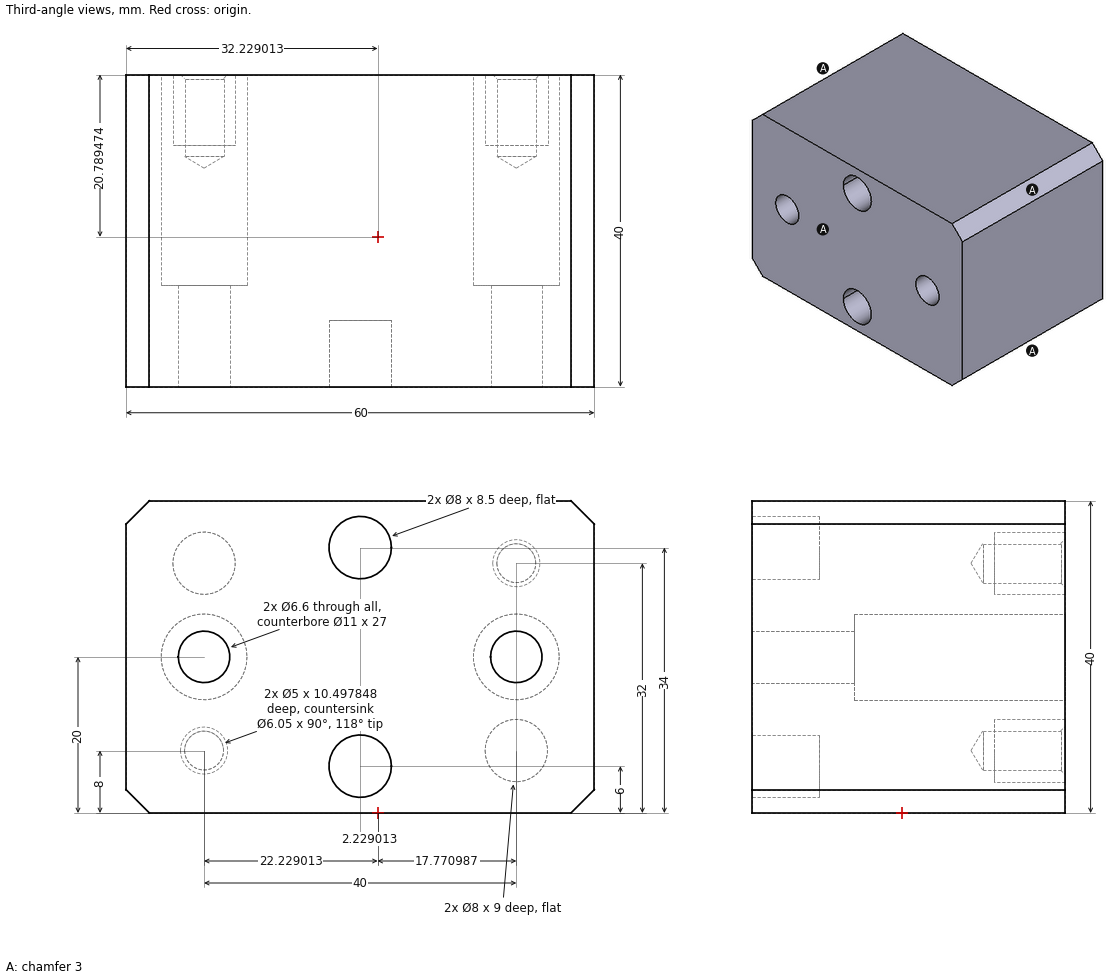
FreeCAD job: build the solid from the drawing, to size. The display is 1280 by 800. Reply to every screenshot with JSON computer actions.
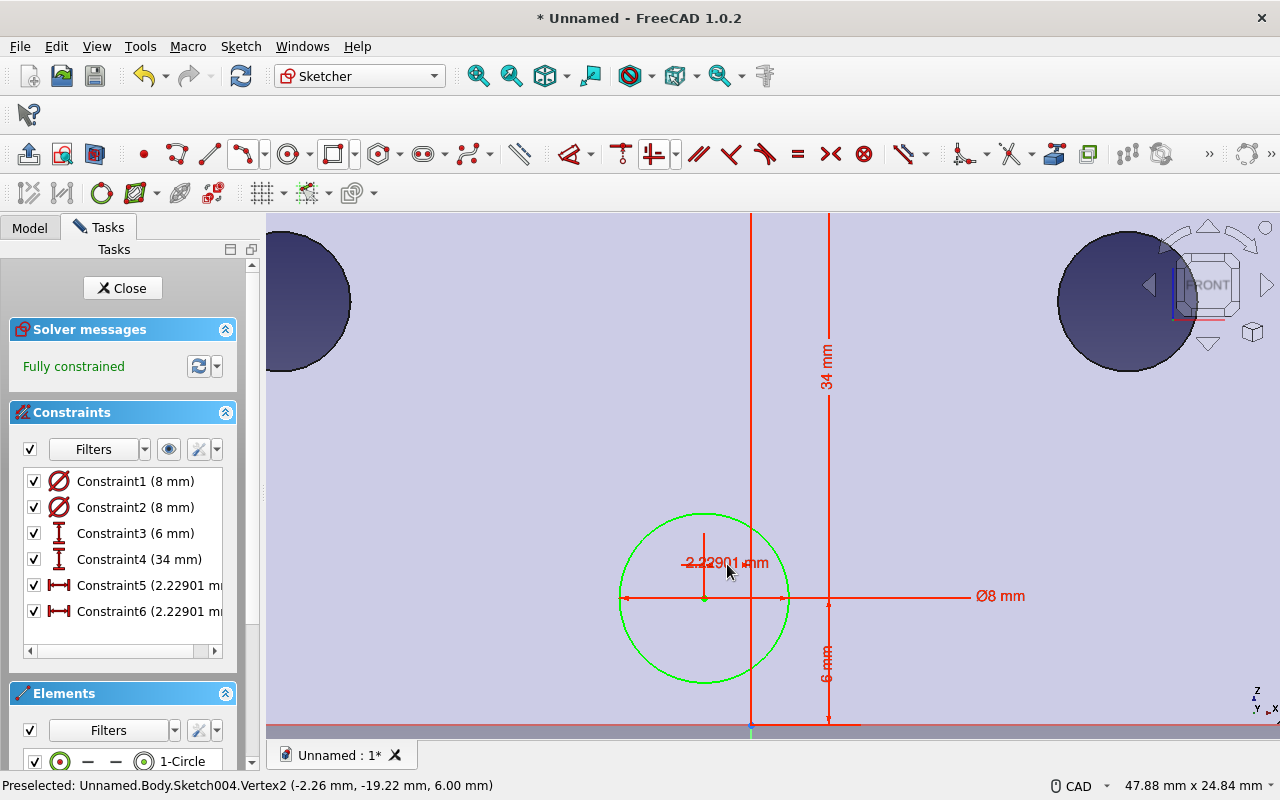
{"action": "left_click", "coordinate": [123, 288]}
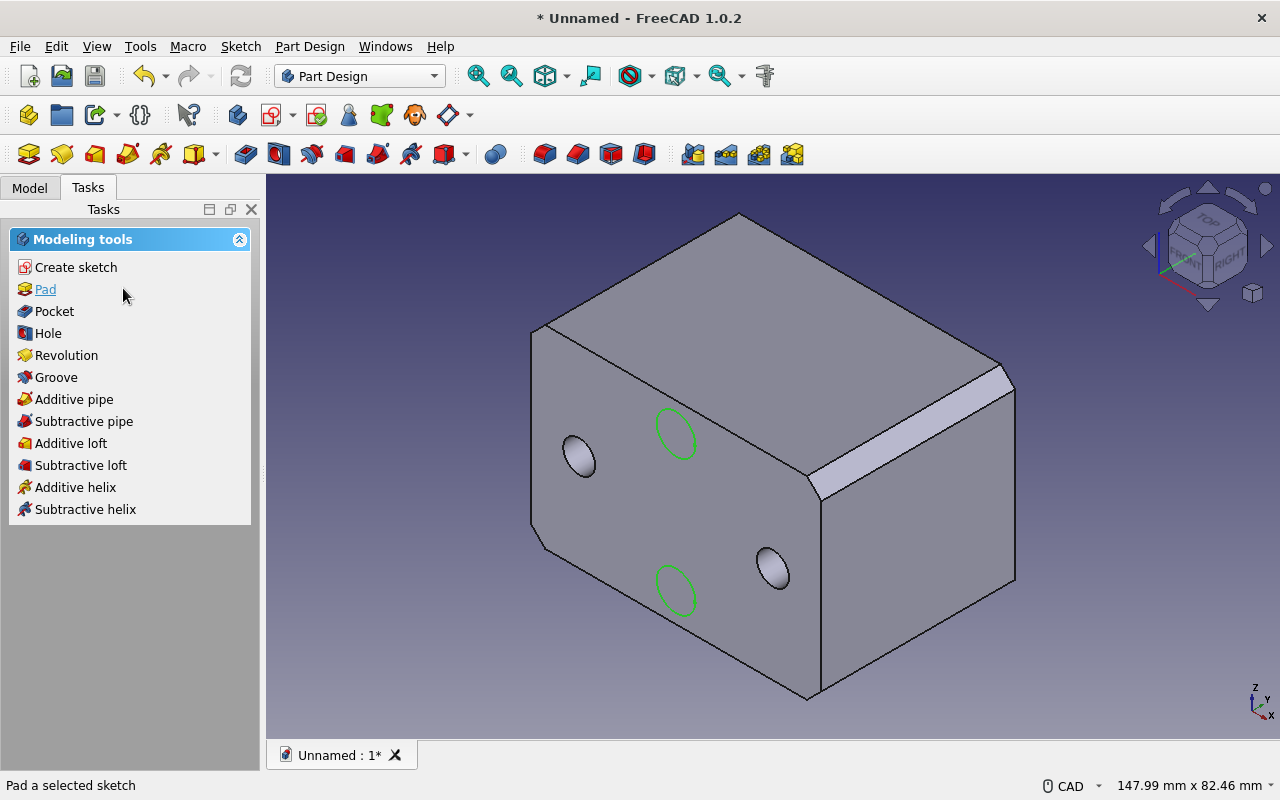
{"action": "left_click", "coordinate": [279, 154]}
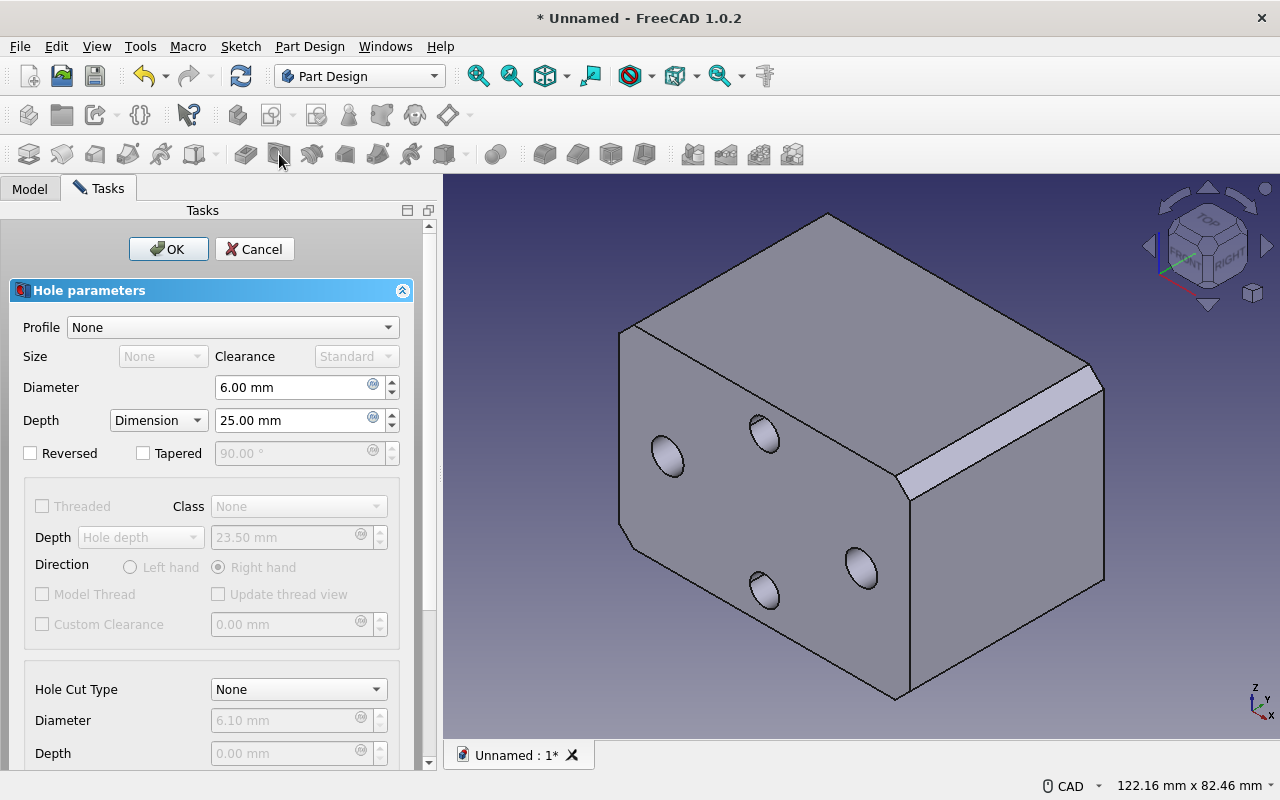
{"action": "triple_click", "coordinate": [300, 388]}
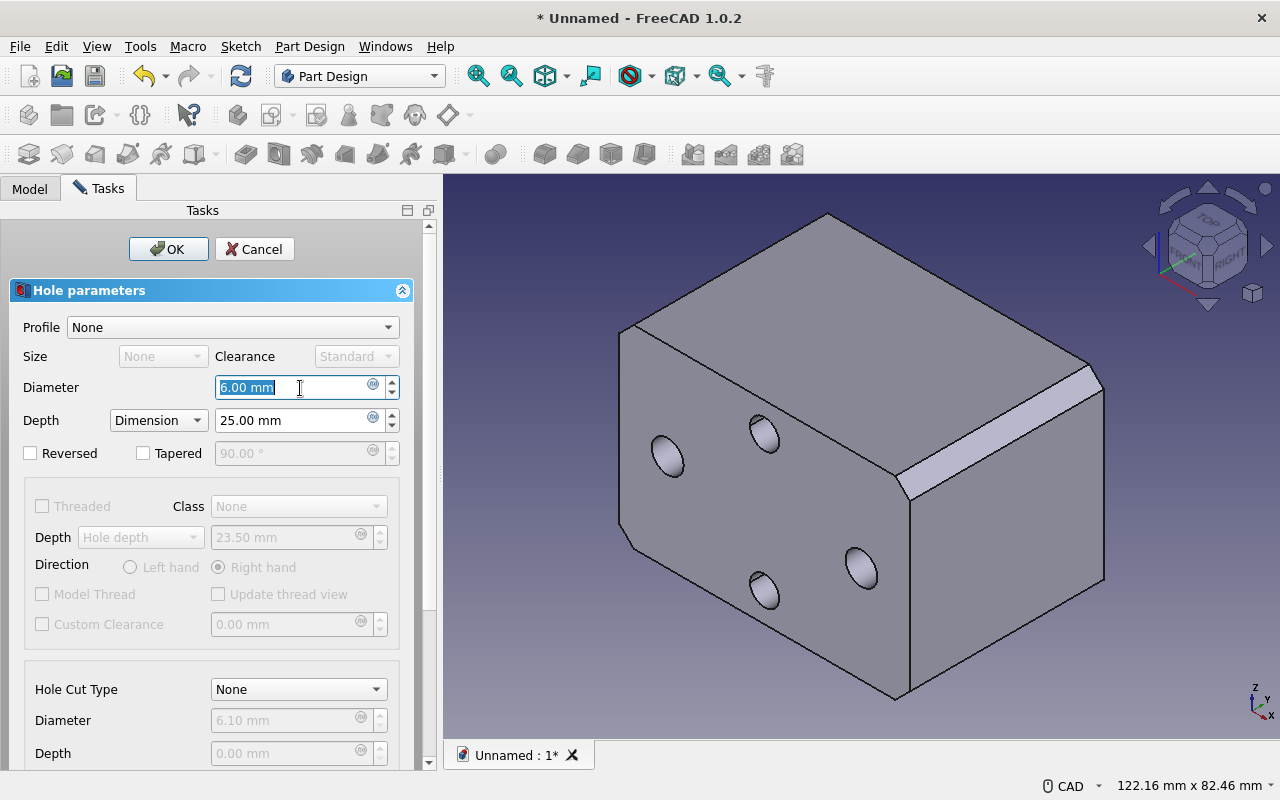
{"action": "type", "text": "8"}
{"action": "key", "text": "Tab"}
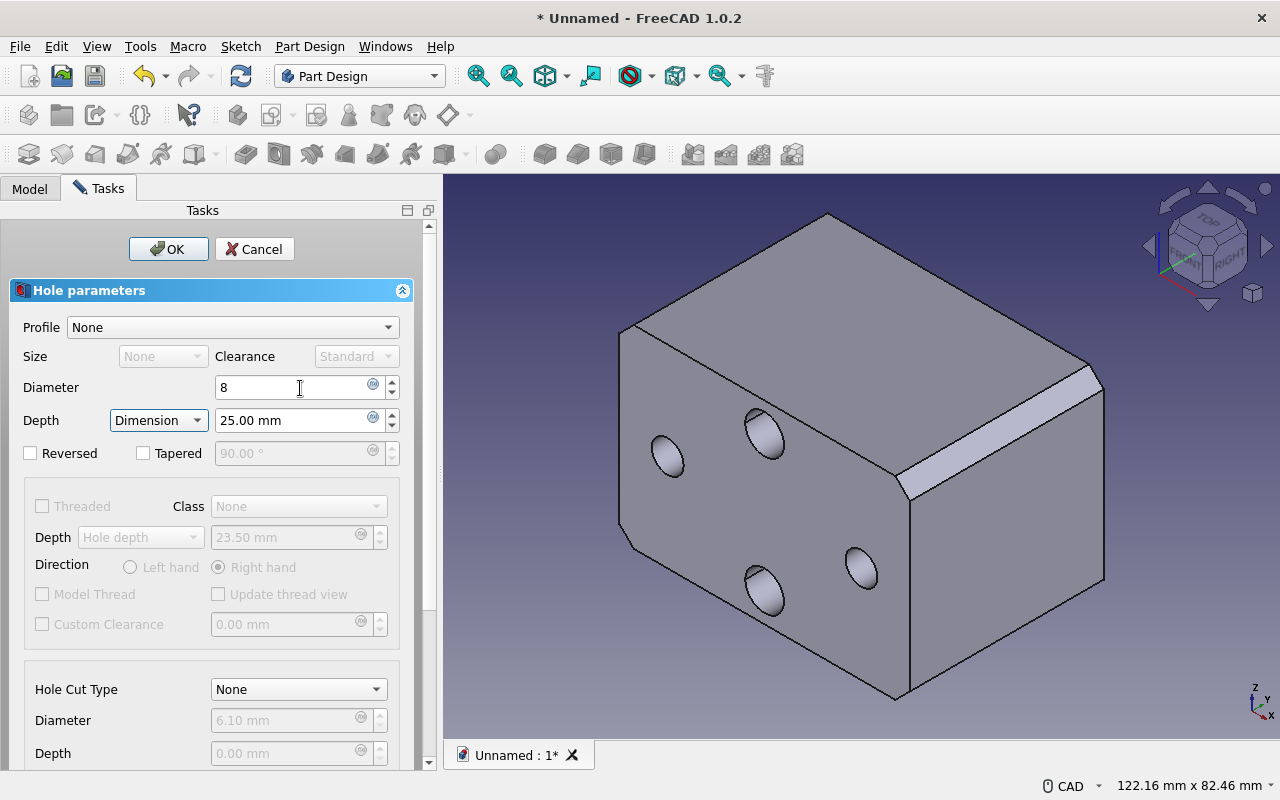
{"action": "triple_click", "coordinate": [300, 420]}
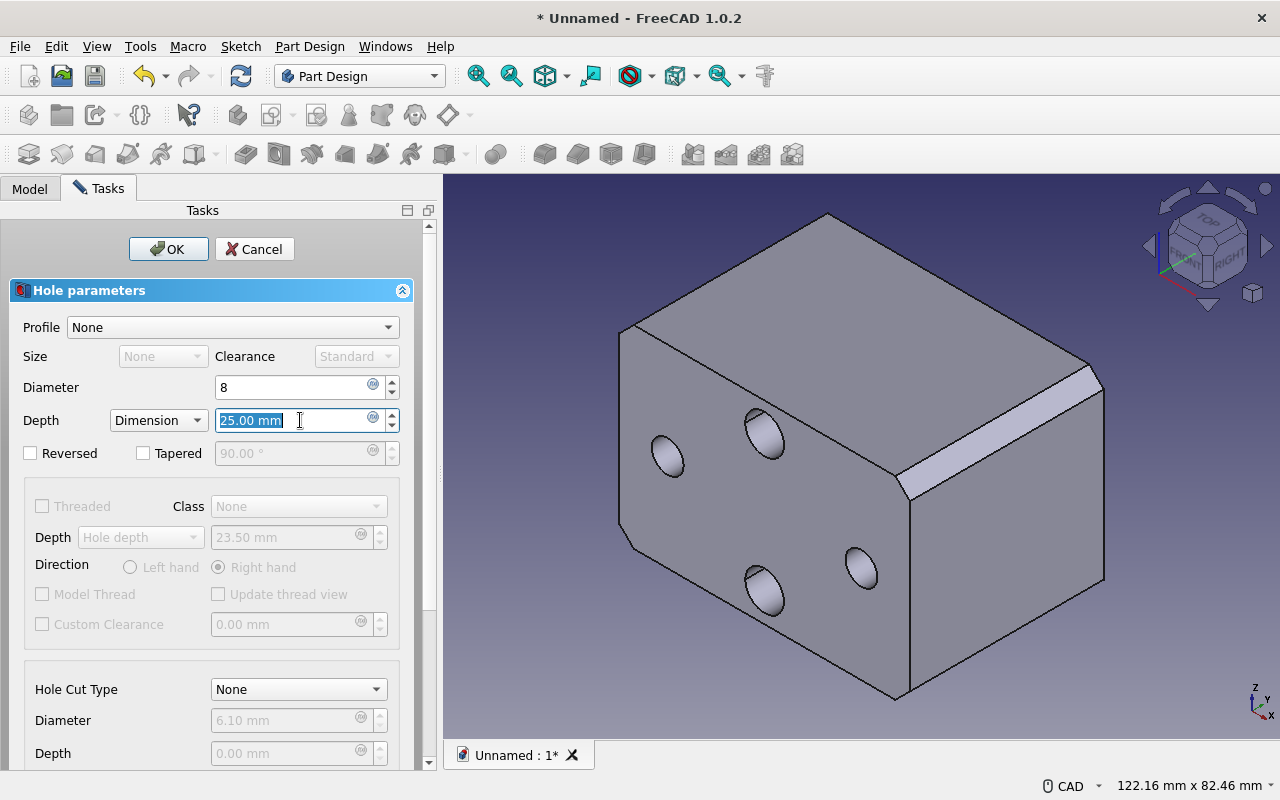
{"action": "type", "text": "8.5"}
{"action": "key", "text": "Tab"}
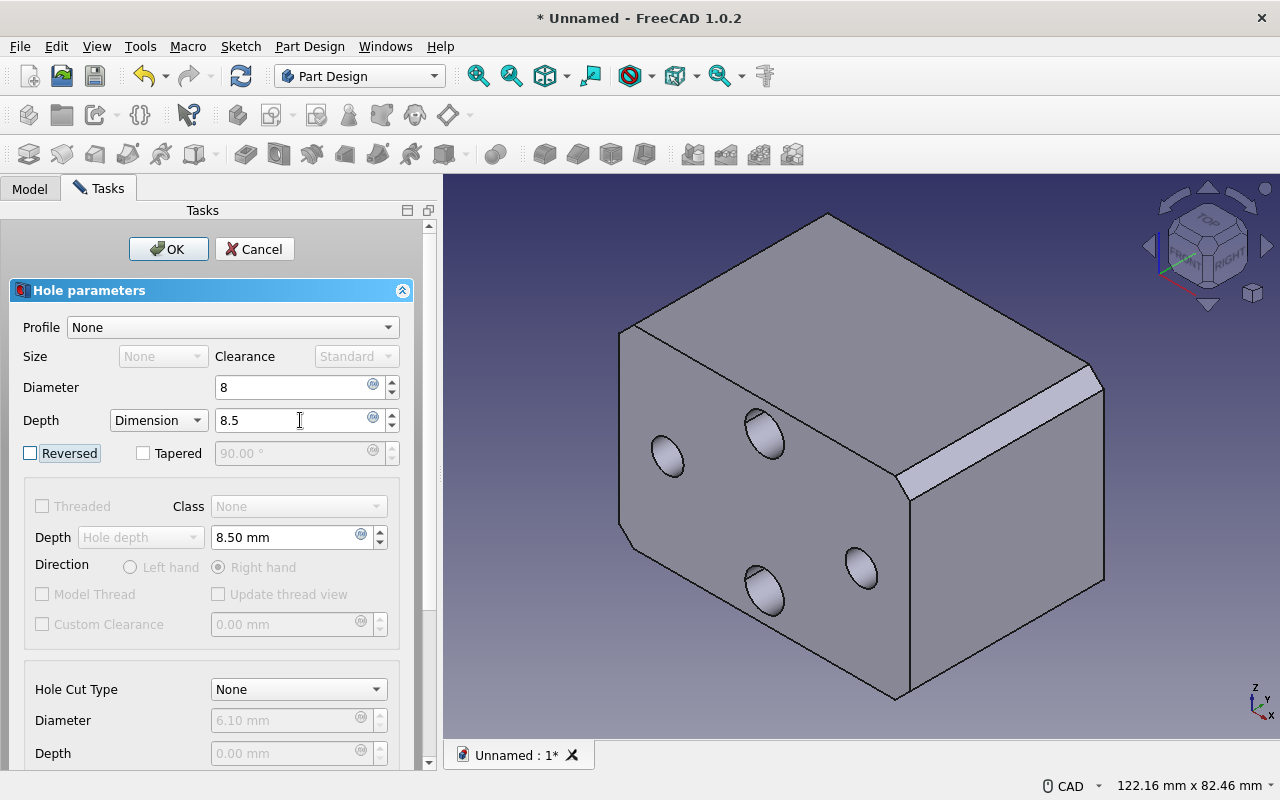
{"action": "scroll", "coordinate": [429, 495], "scroll_direction": "down", "scroll_amount": 3}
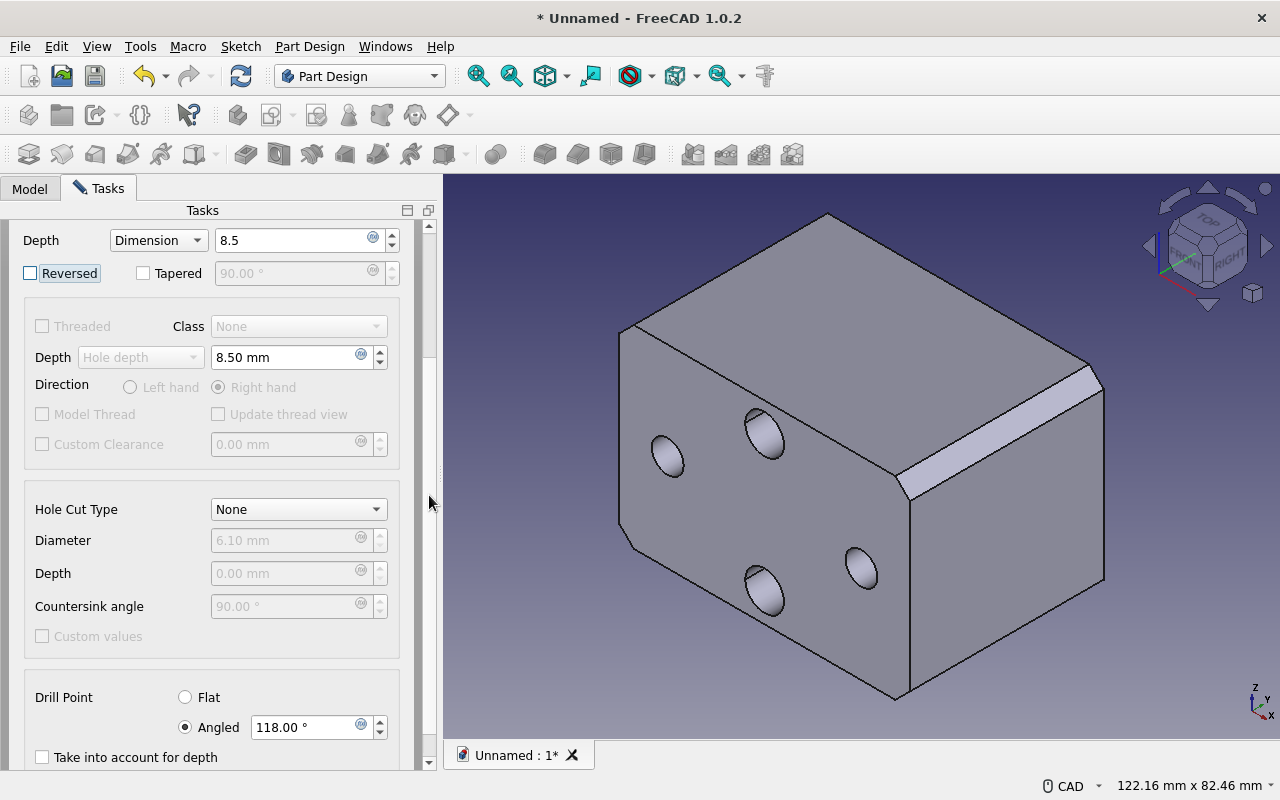
{"action": "left_click", "coordinate": [186, 695]}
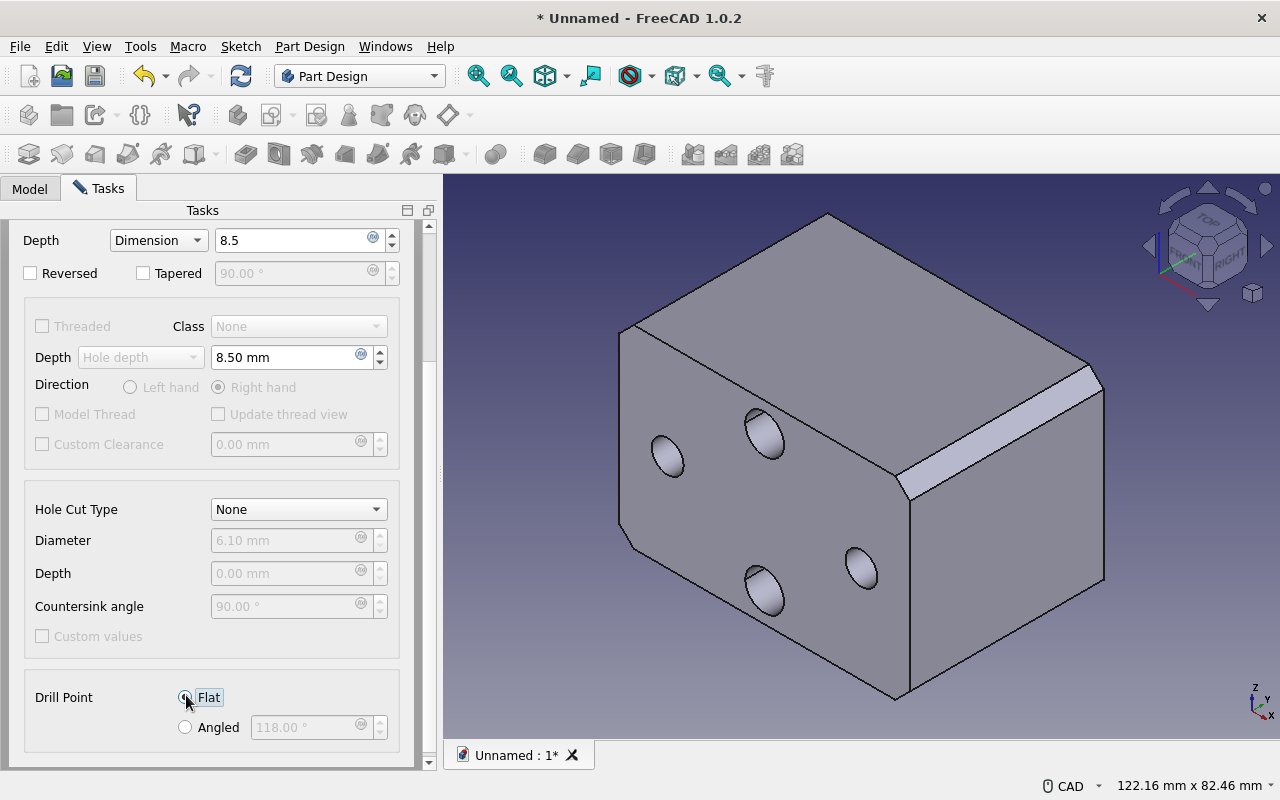
{"action": "scroll", "coordinate": [429, 495], "scroll_direction": "up", "scroll_amount": 4}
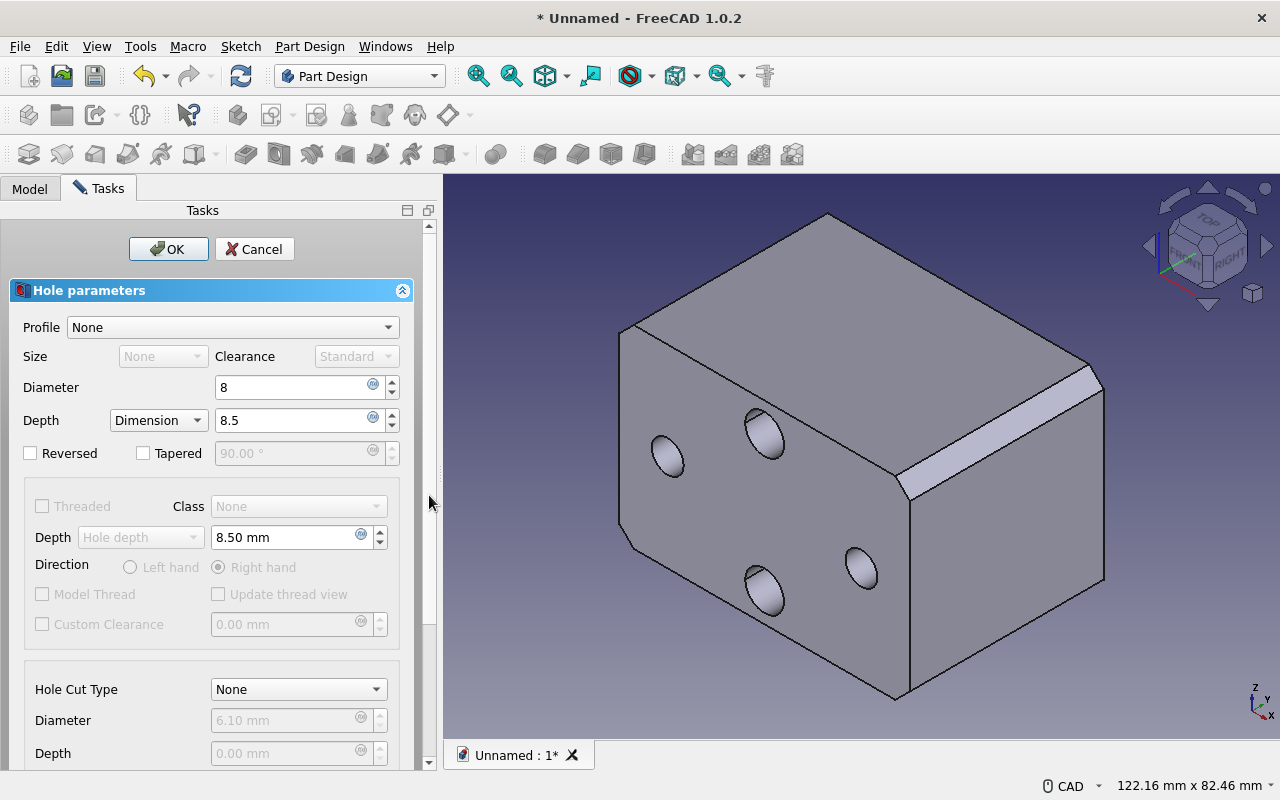
{"action": "left_click", "coordinate": [169, 249]}